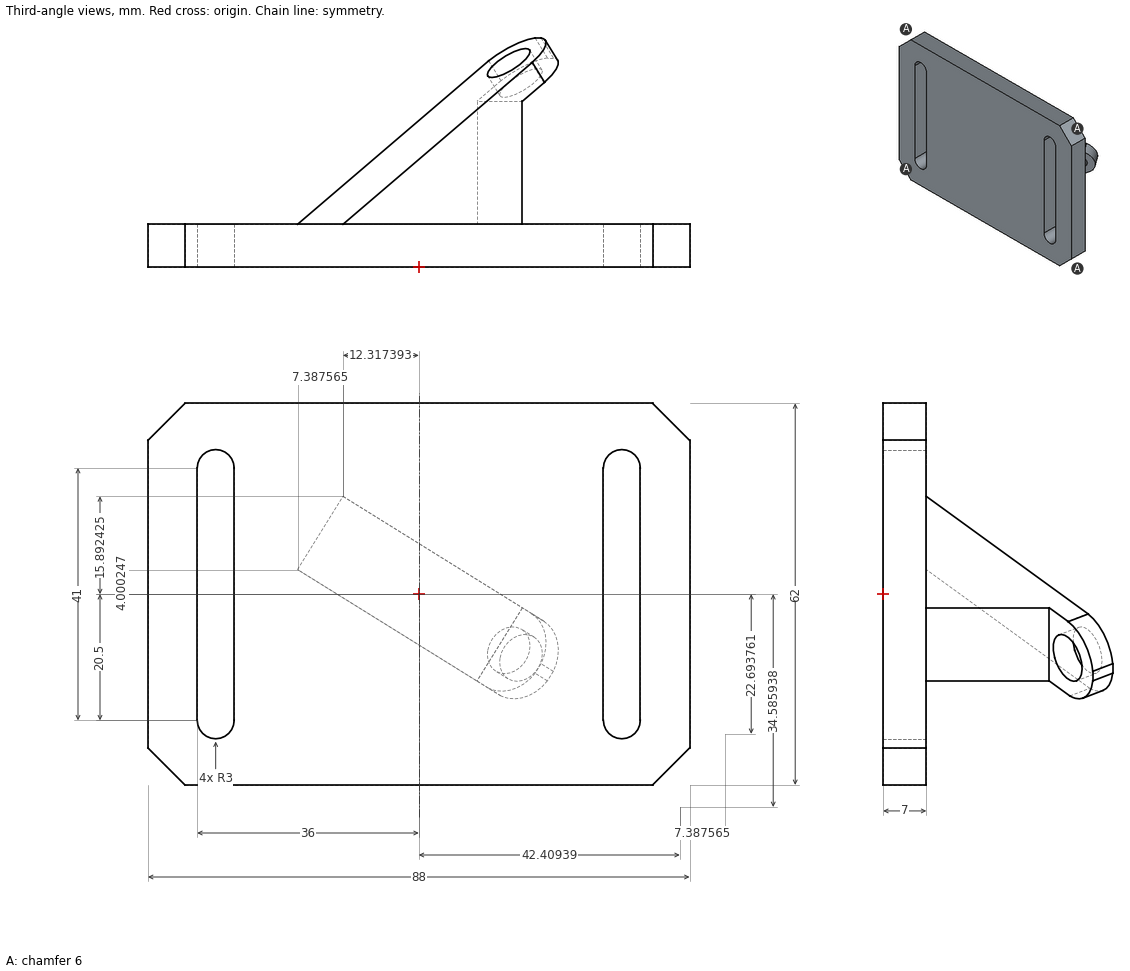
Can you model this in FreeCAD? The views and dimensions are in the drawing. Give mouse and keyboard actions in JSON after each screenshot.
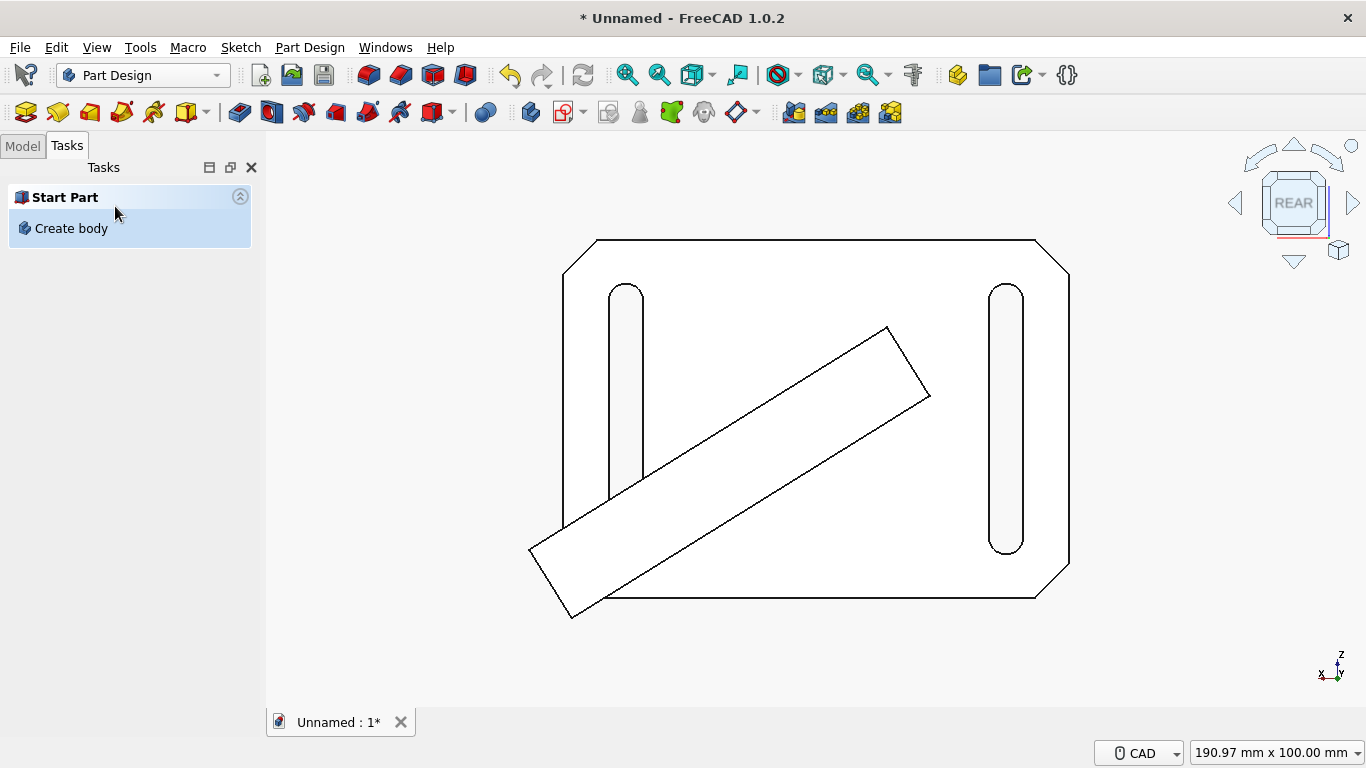
{"action": "key", "text": "0"}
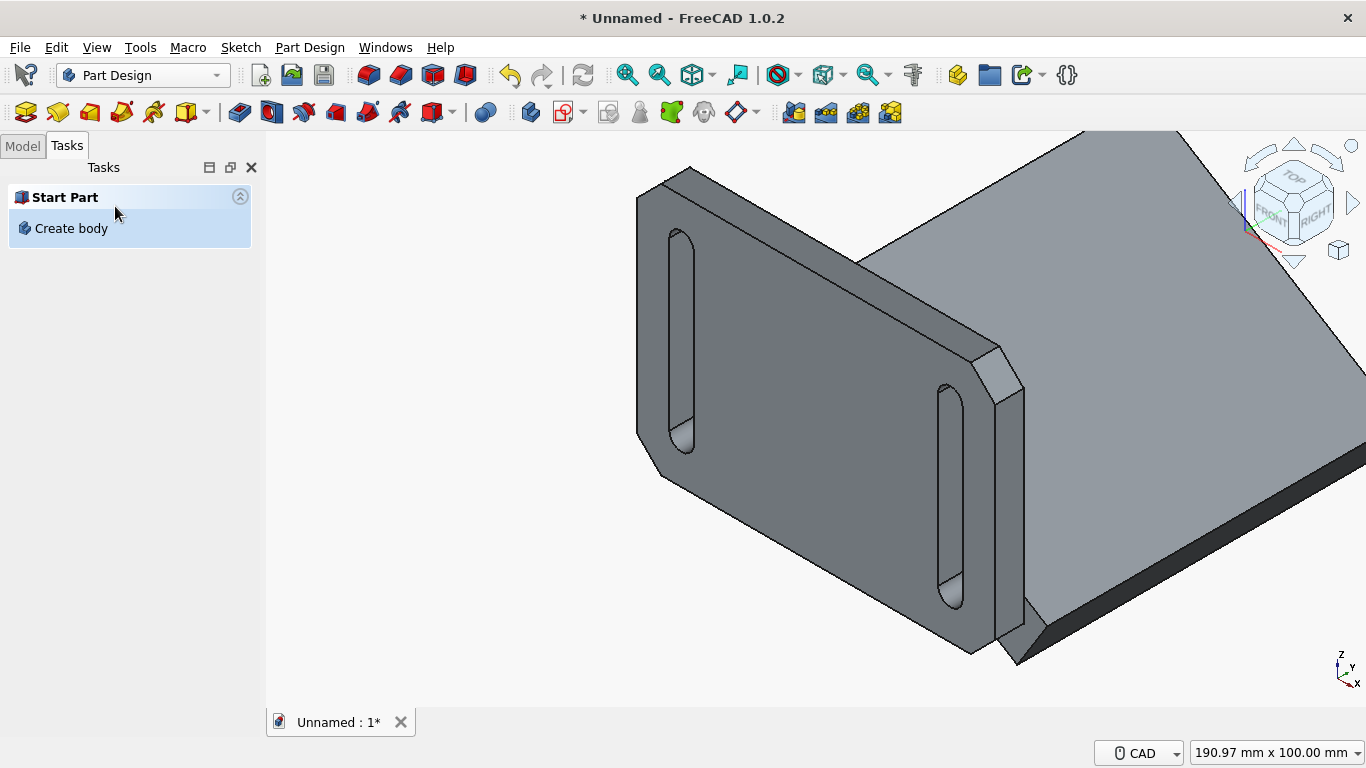
{"action": "left_click", "coordinate": [628, 76]}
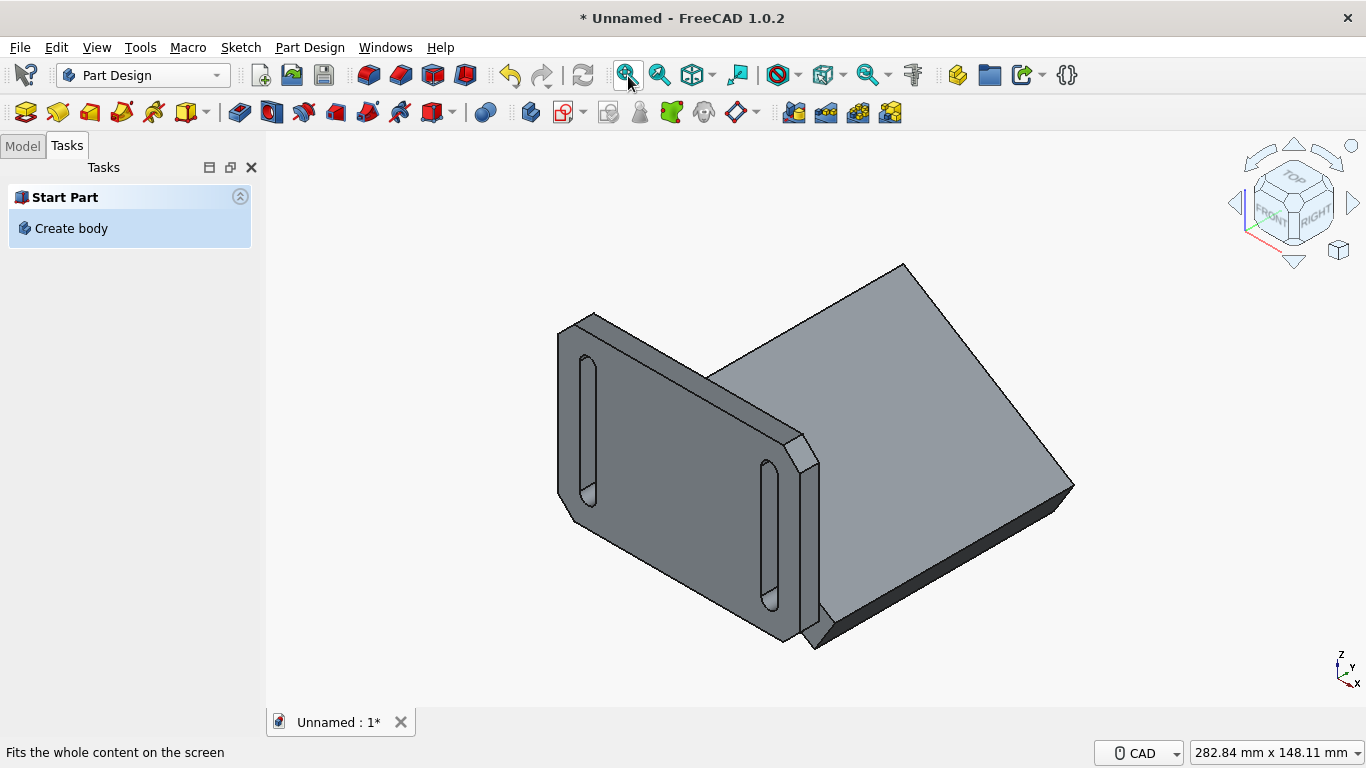
{"action": "left_click", "coordinate": [869, 443]}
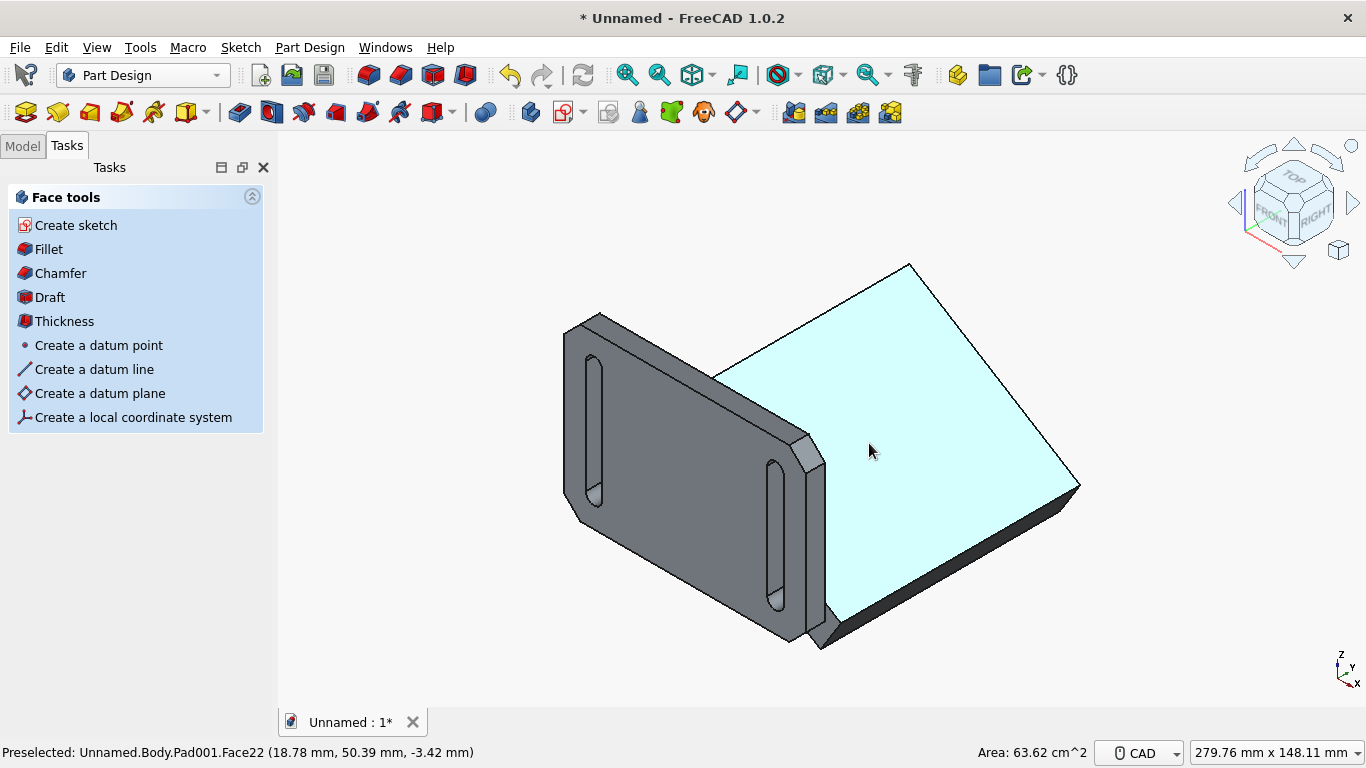
{"action": "left_click", "coordinate": [564, 112]}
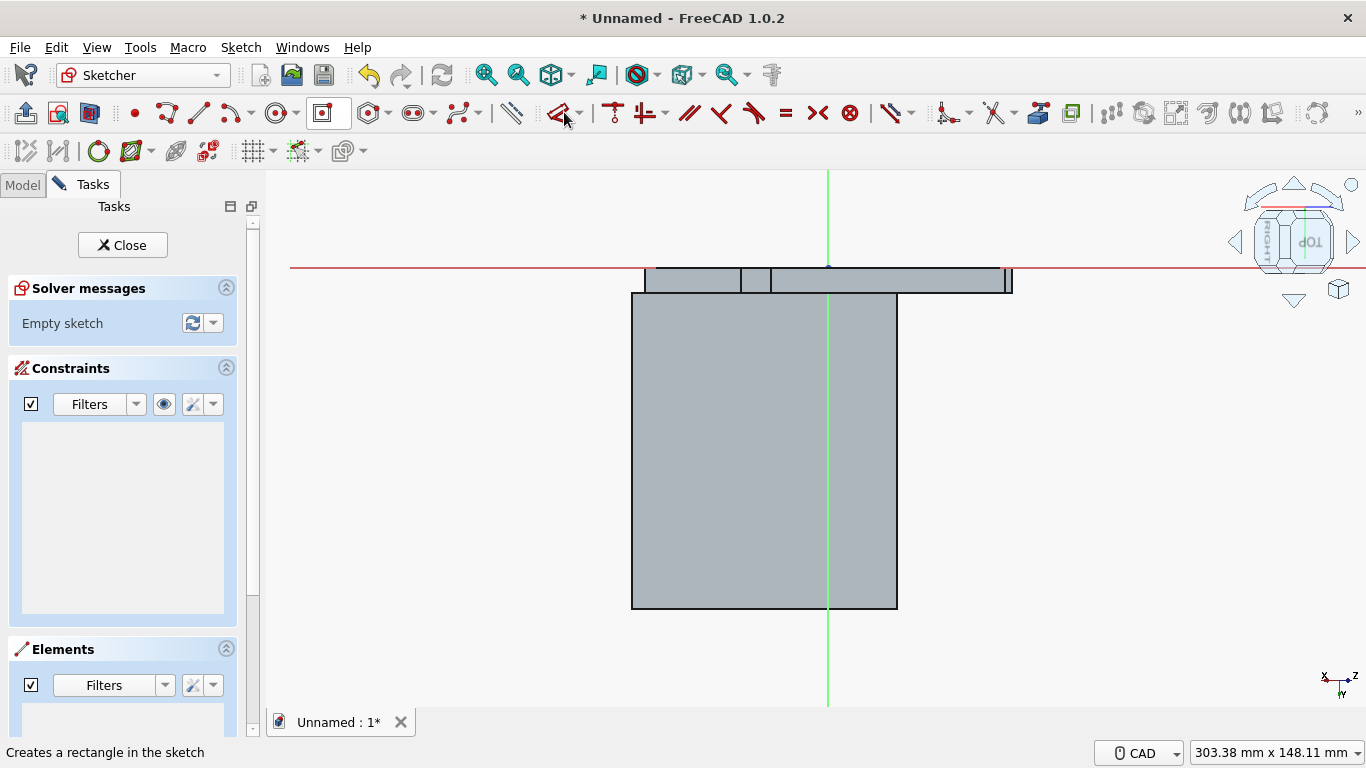
{"action": "left_click", "coordinate": [90, 114]}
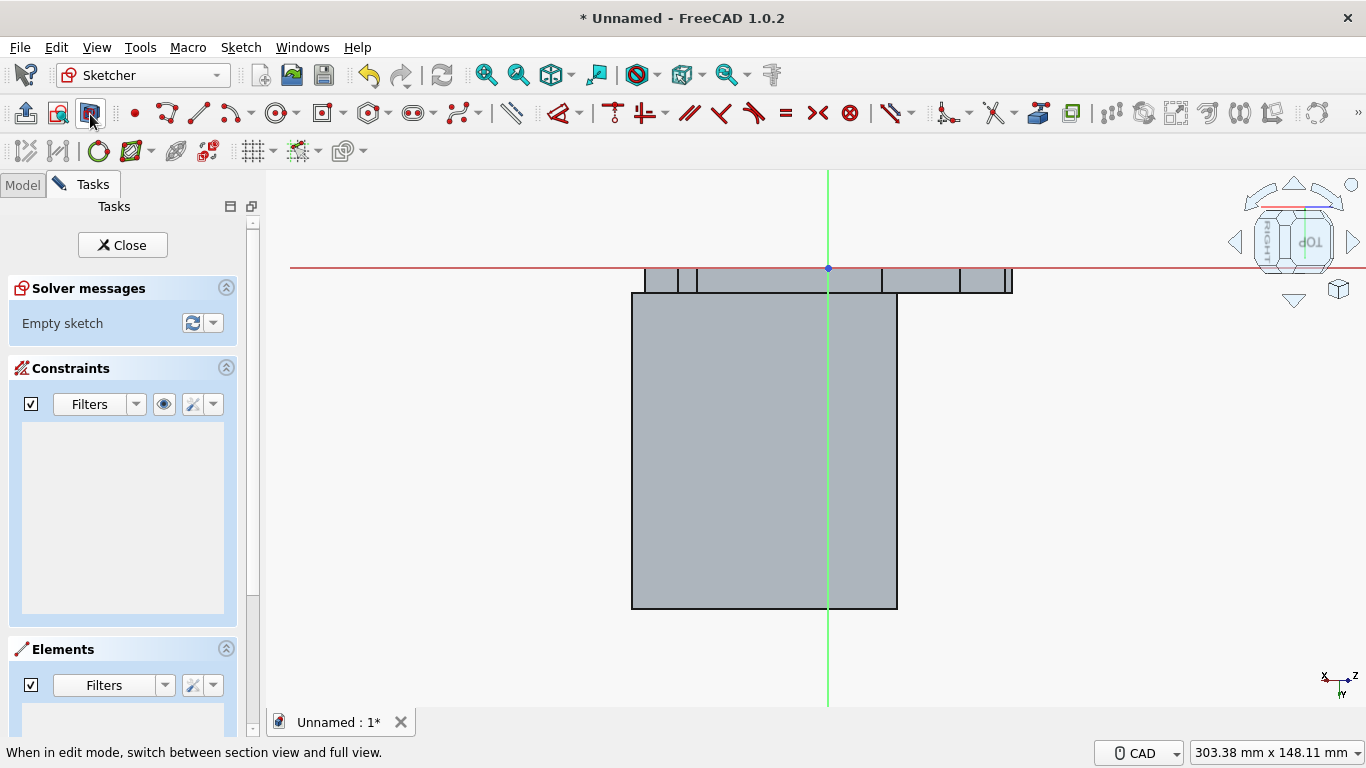
{"action": "scroll", "coordinate": [491, 335], "scroll_direction": "down", "scroll_amount": 1}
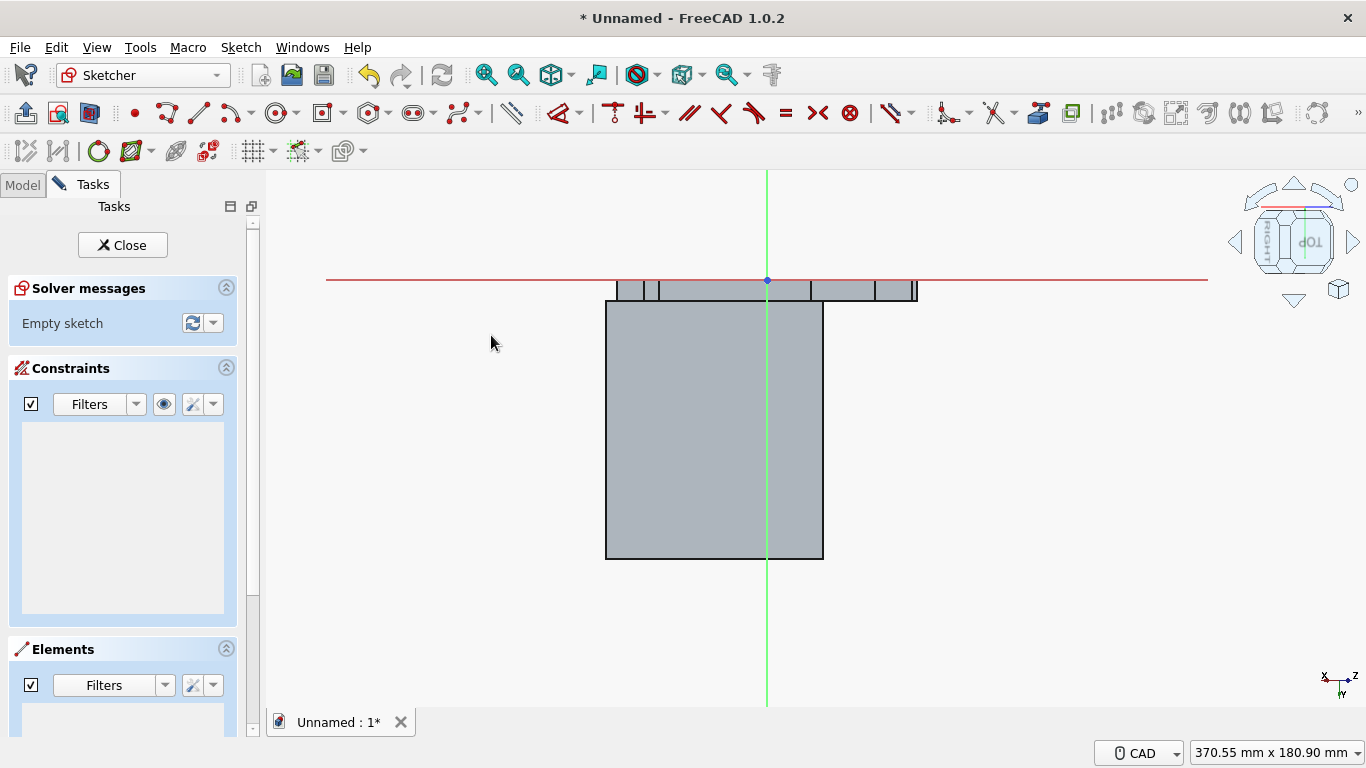
{"action": "left_click", "coordinate": [168, 114]}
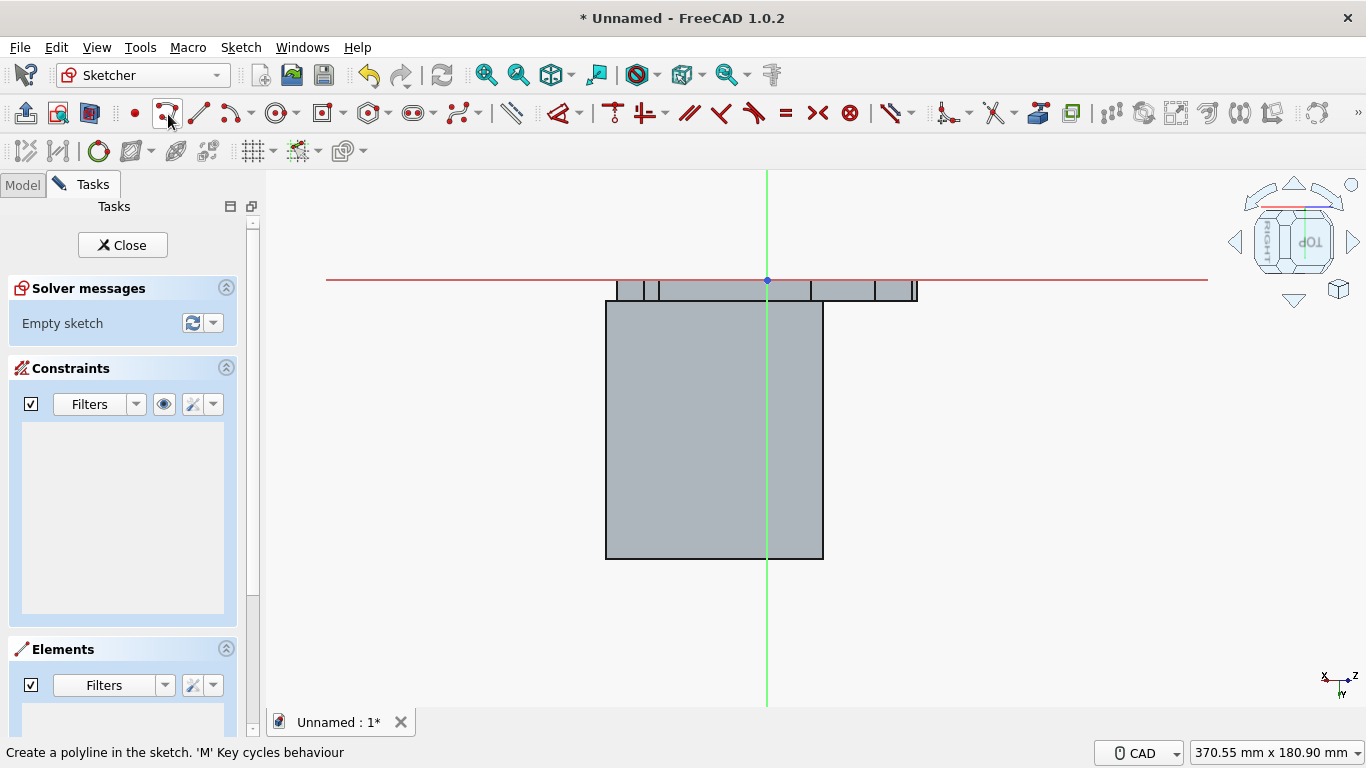
{"action": "left_click", "coordinate": [721, 301]}
{"action": "left_click", "coordinate": [586, 301]}
{"action": "left_click", "coordinate": [457, 416]}
{"action": "left_click", "coordinate": [465, 557]}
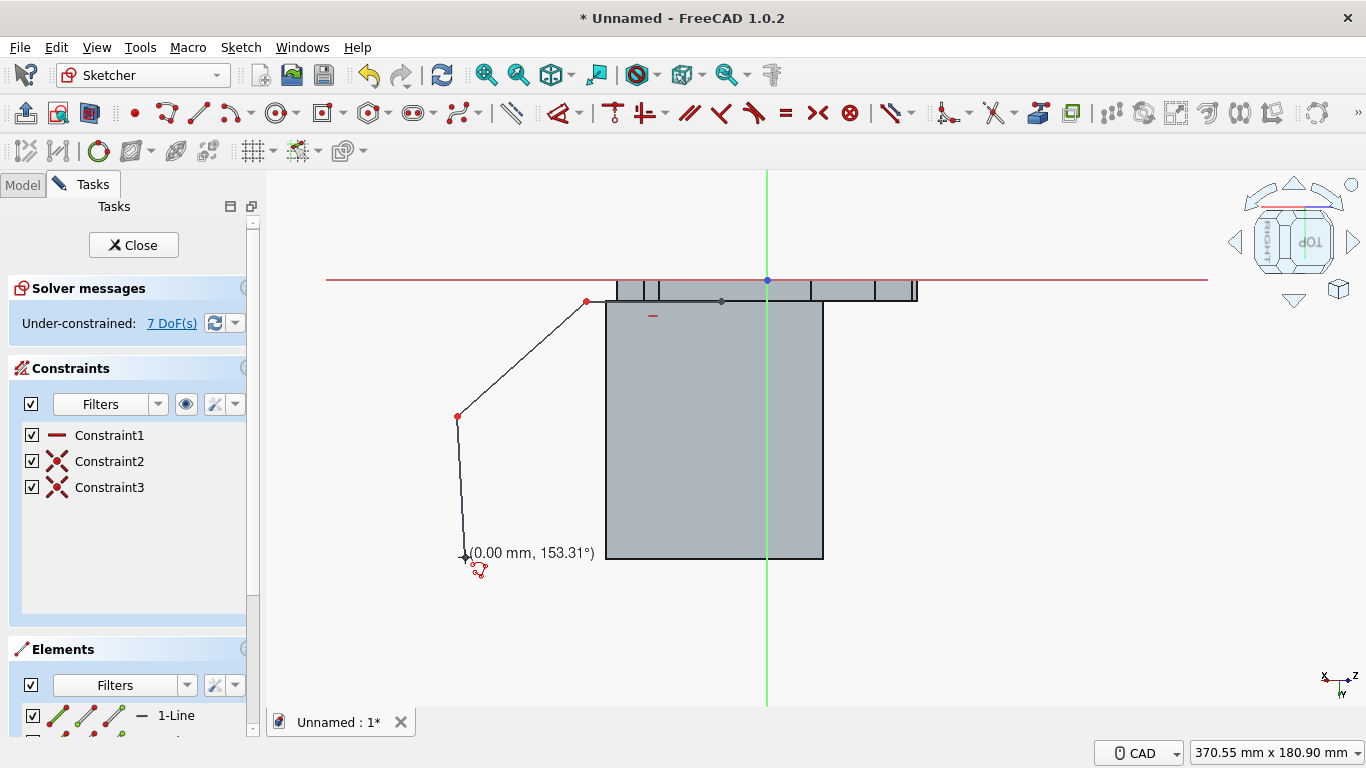
{"action": "scroll", "coordinate": [776, 597], "scroll_direction": "up", "scroll_amount": 3}